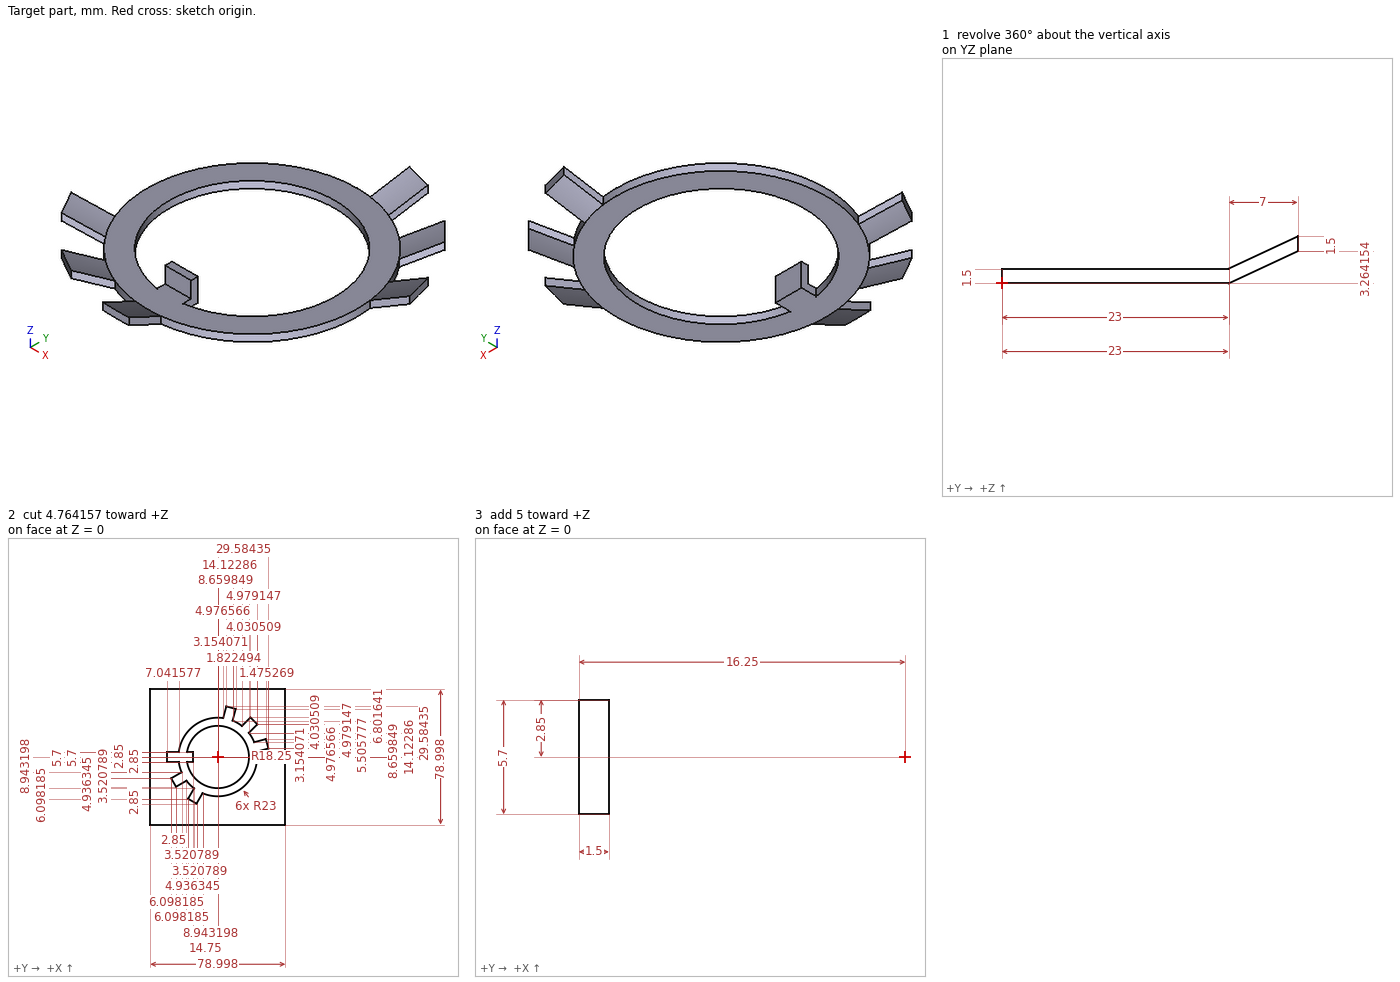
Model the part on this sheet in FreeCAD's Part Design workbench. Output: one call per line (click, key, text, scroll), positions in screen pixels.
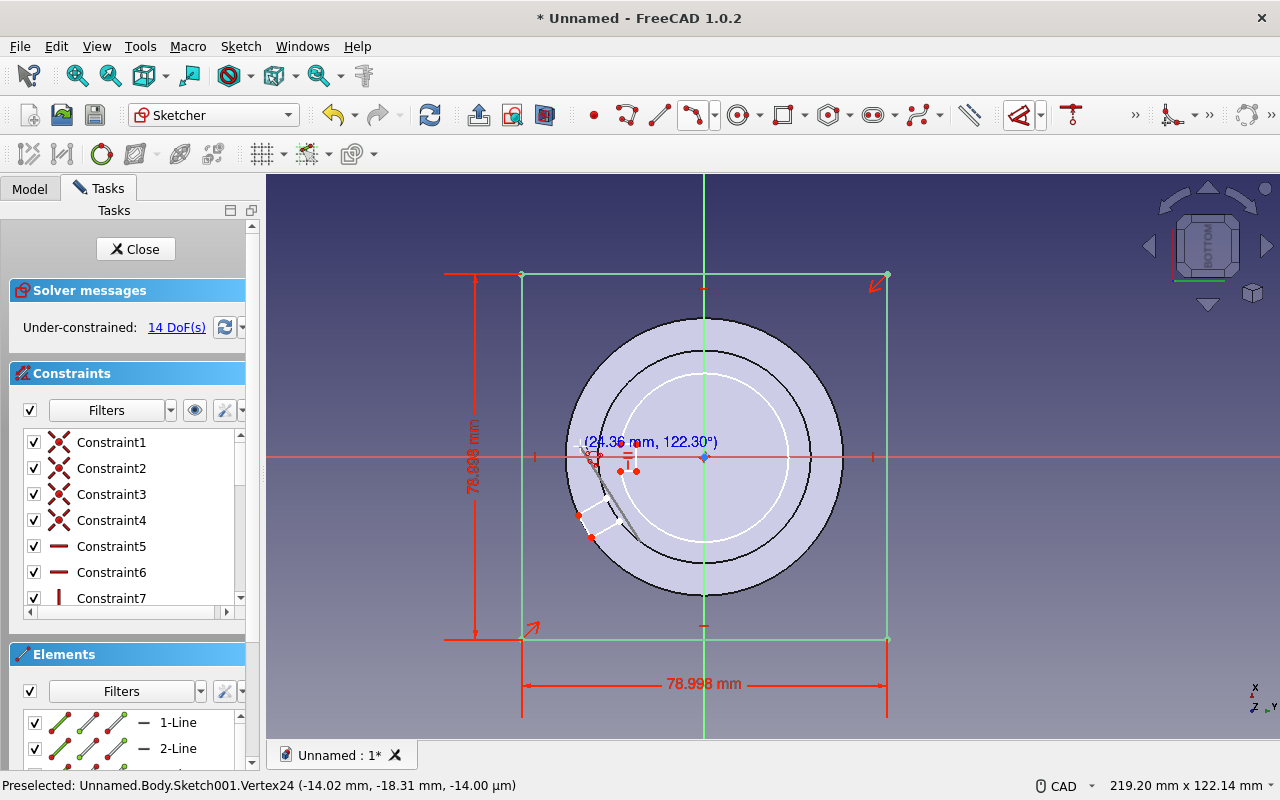
click(624, 570)
click(647, 583)
click(663, 555)
right_click(663, 555)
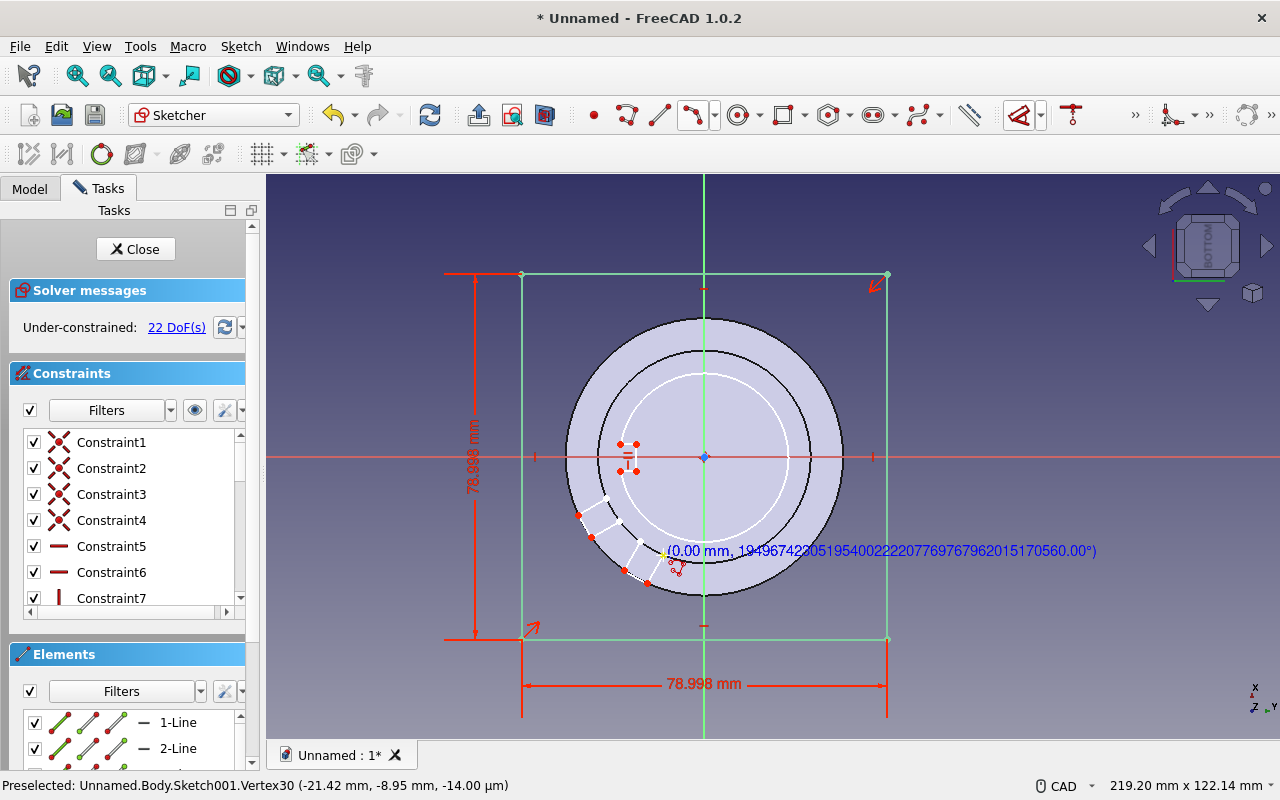
click(810, 442)
click(841, 434)
click(834, 408)
click(803, 417)
right_click(803, 417)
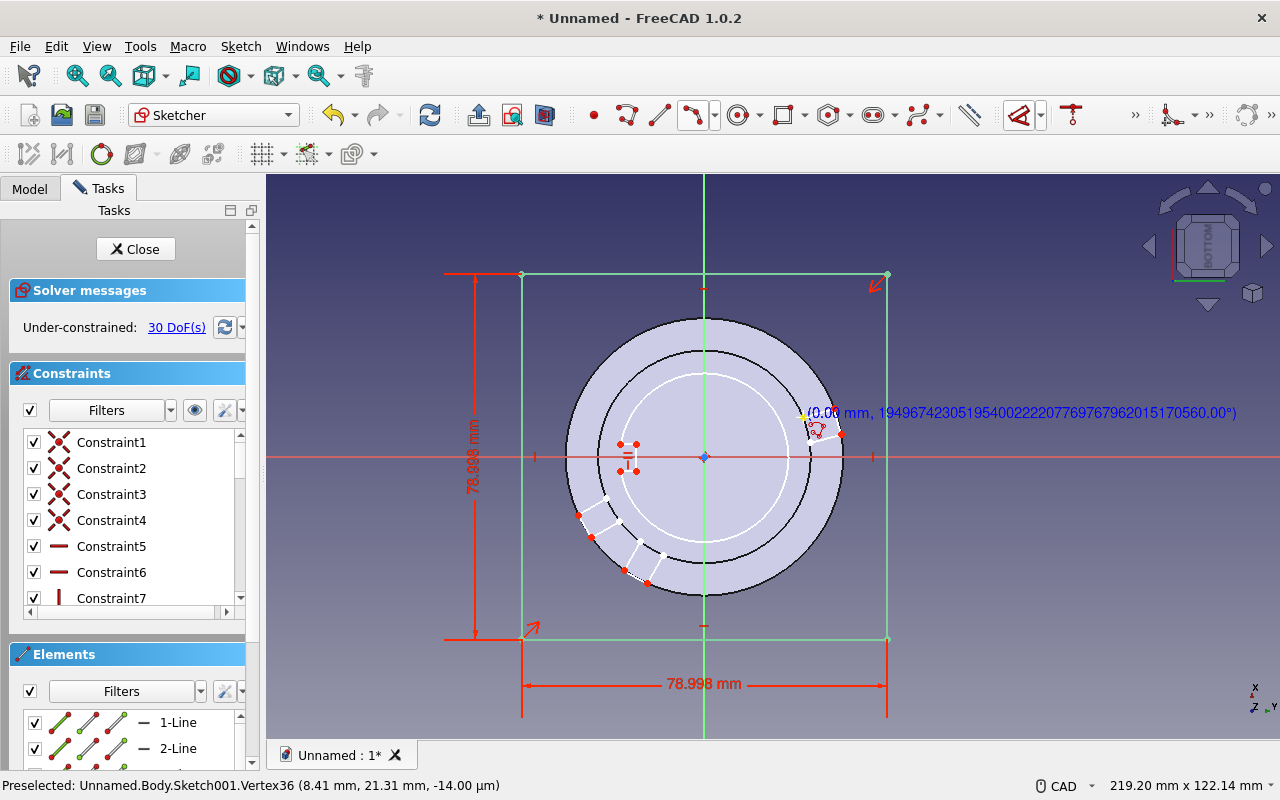
click(788, 392)
click(811, 369)
click(793, 350)
click(770, 373)
right_click(770, 373)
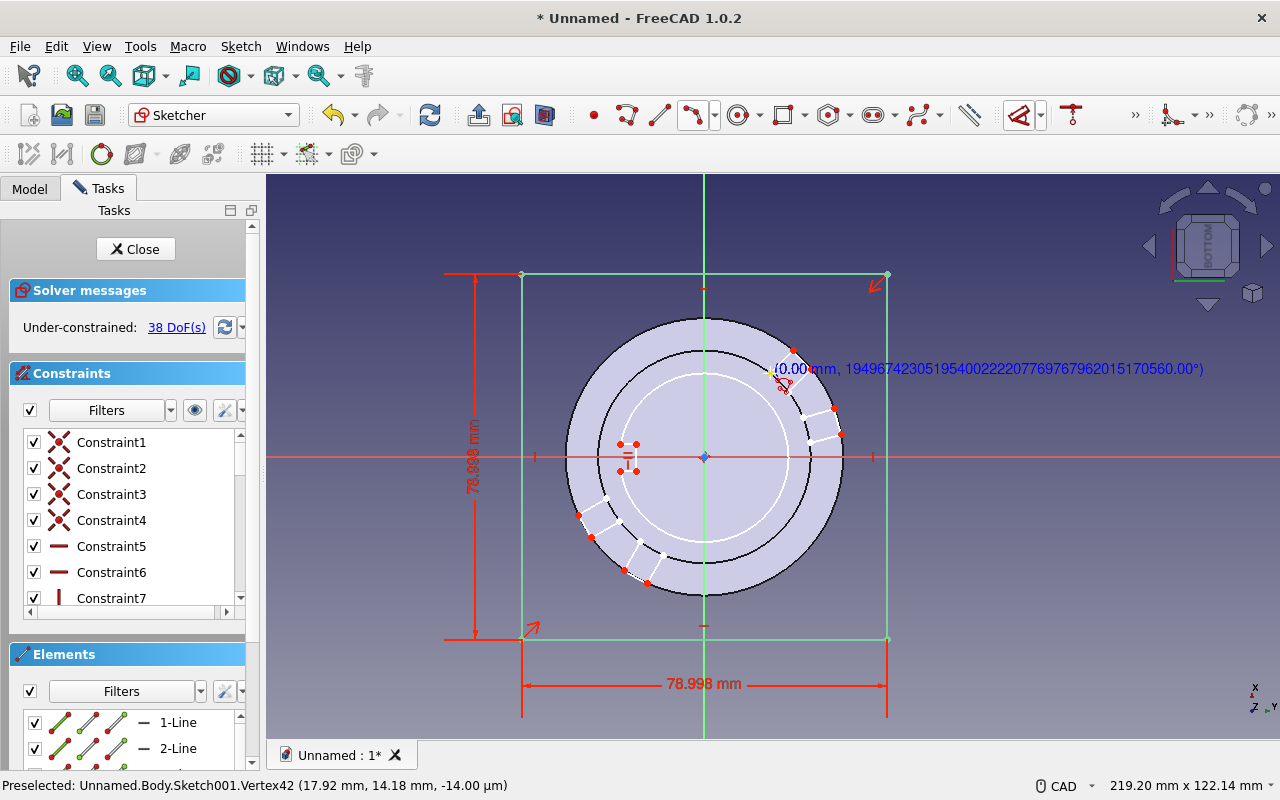
click(744, 358)
click(753, 327)
click(727, 320)
click(719, 352)
right_click(719, 352)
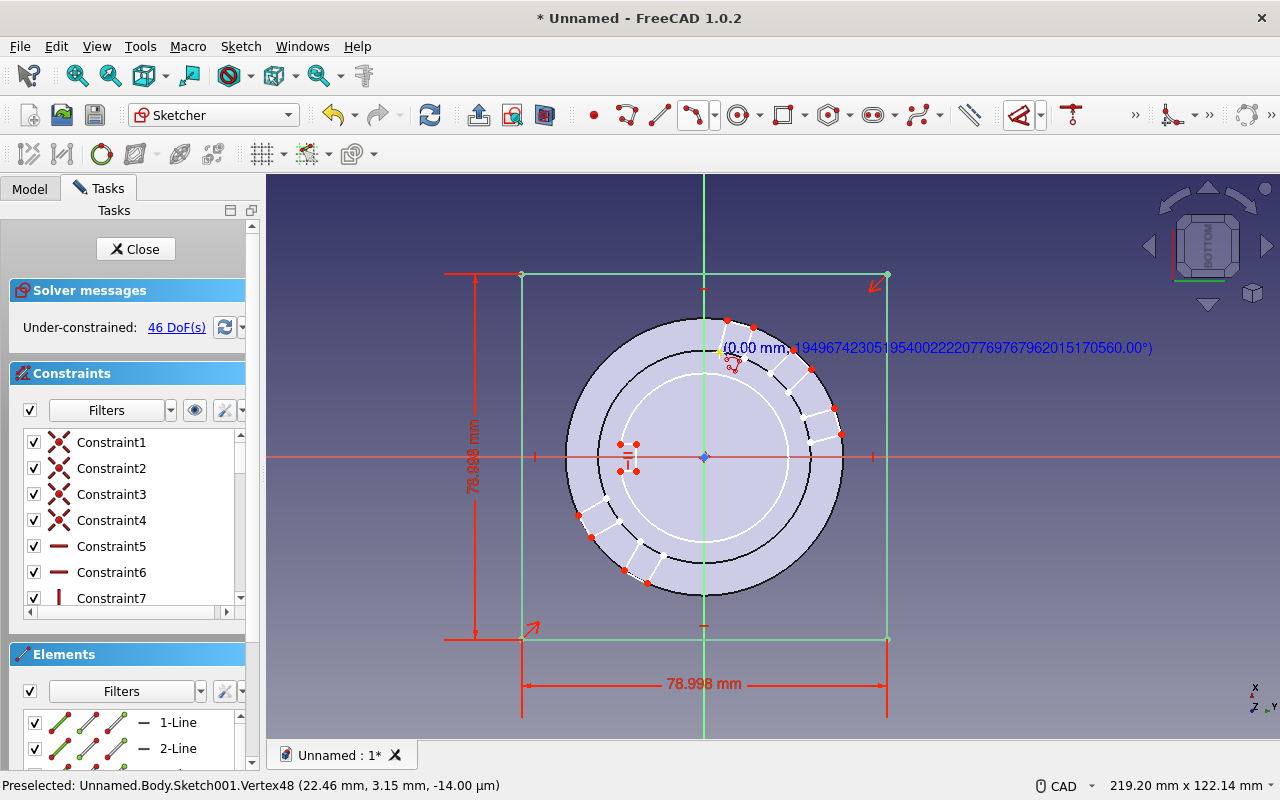
click(599, 444)
click(566, 444)
click(566, 470)
click(599, 470)
right_click(599, 470)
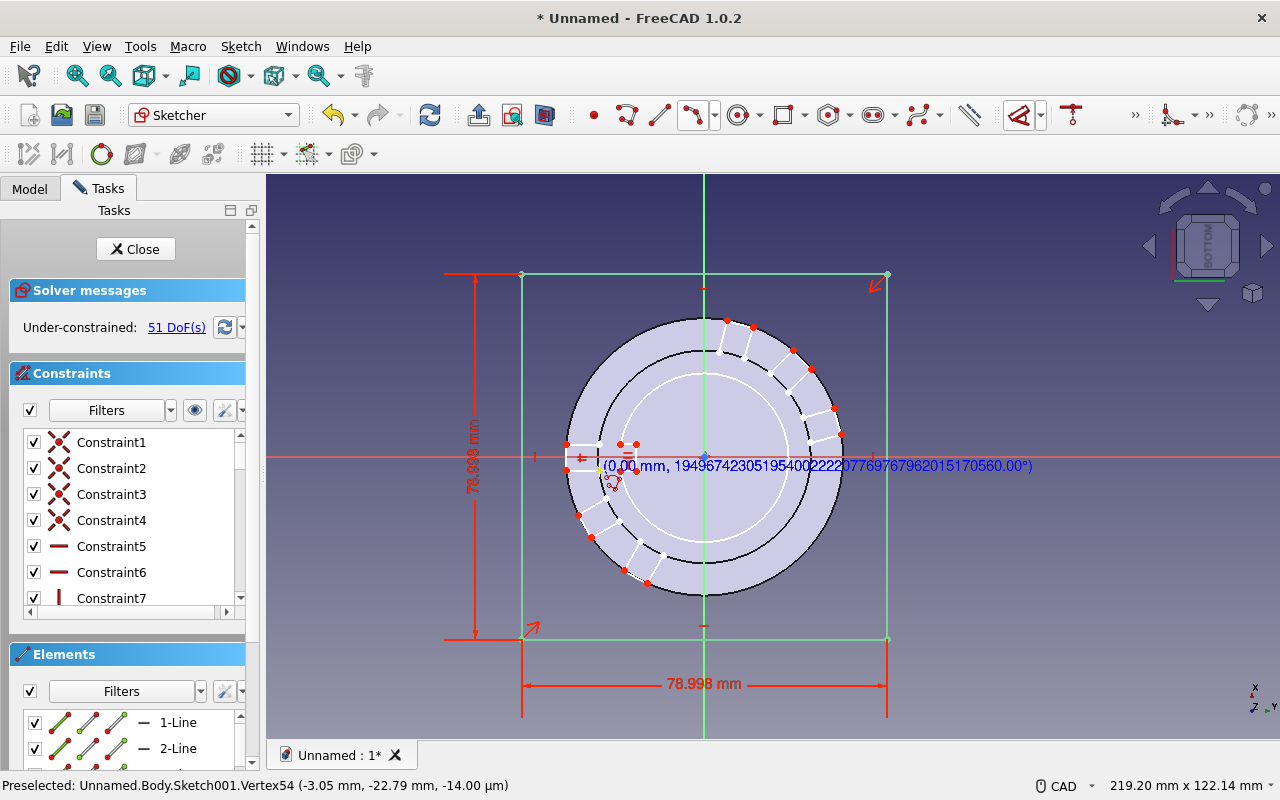
click(692, 116)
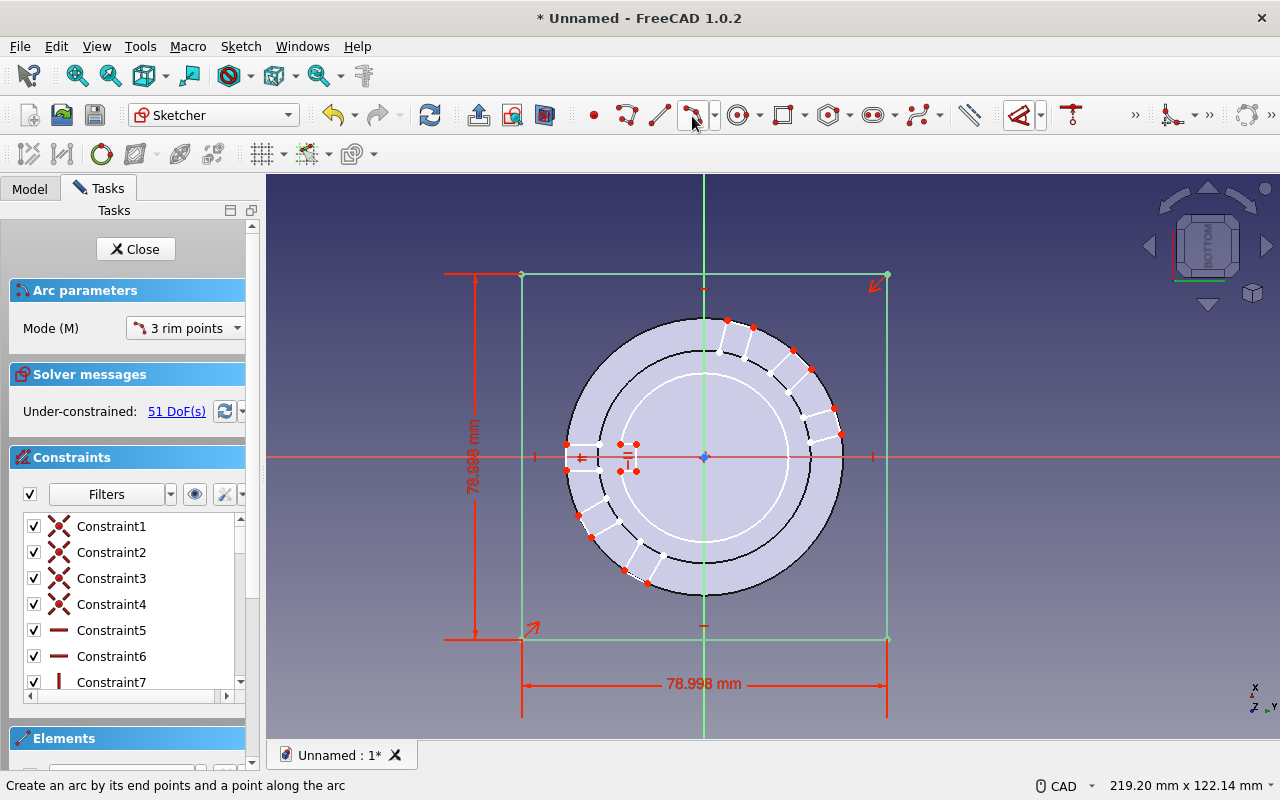
click(620, 522)
click(640, 542)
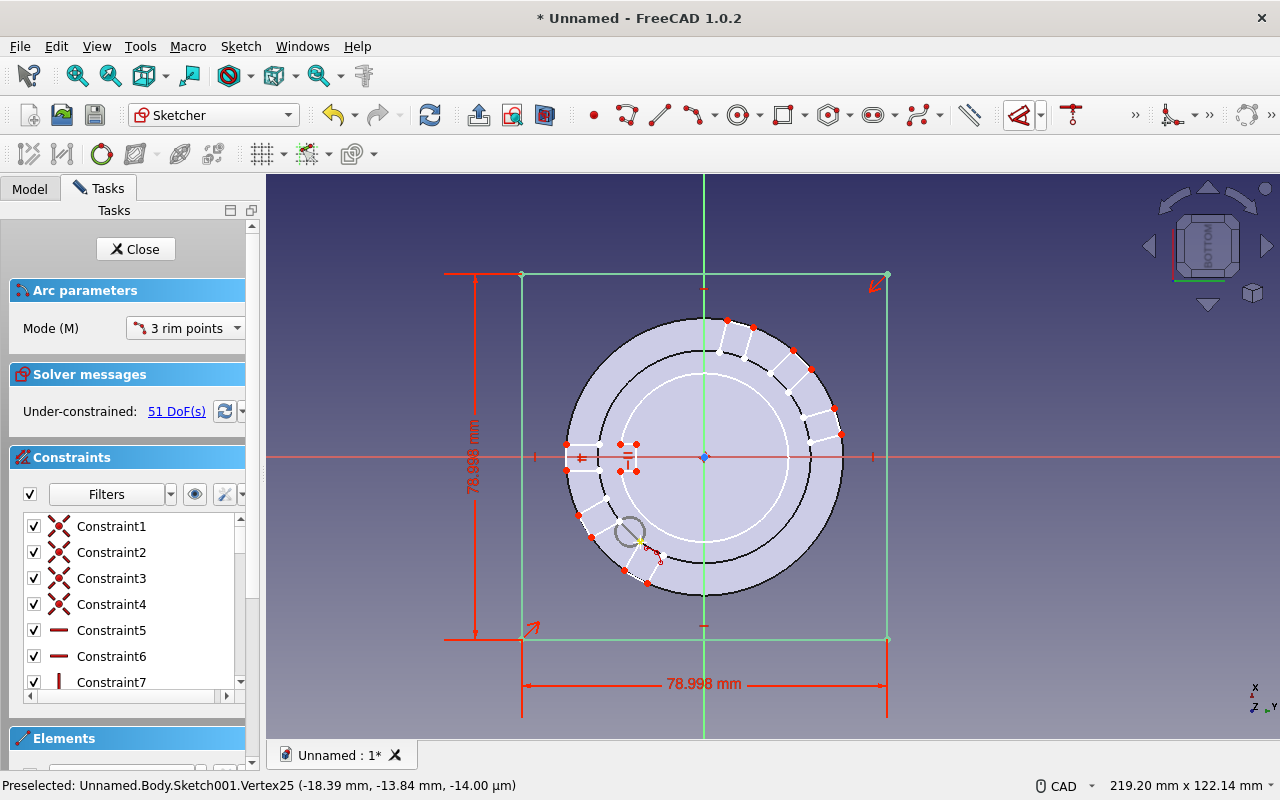
scroll(629, 532, up, 14)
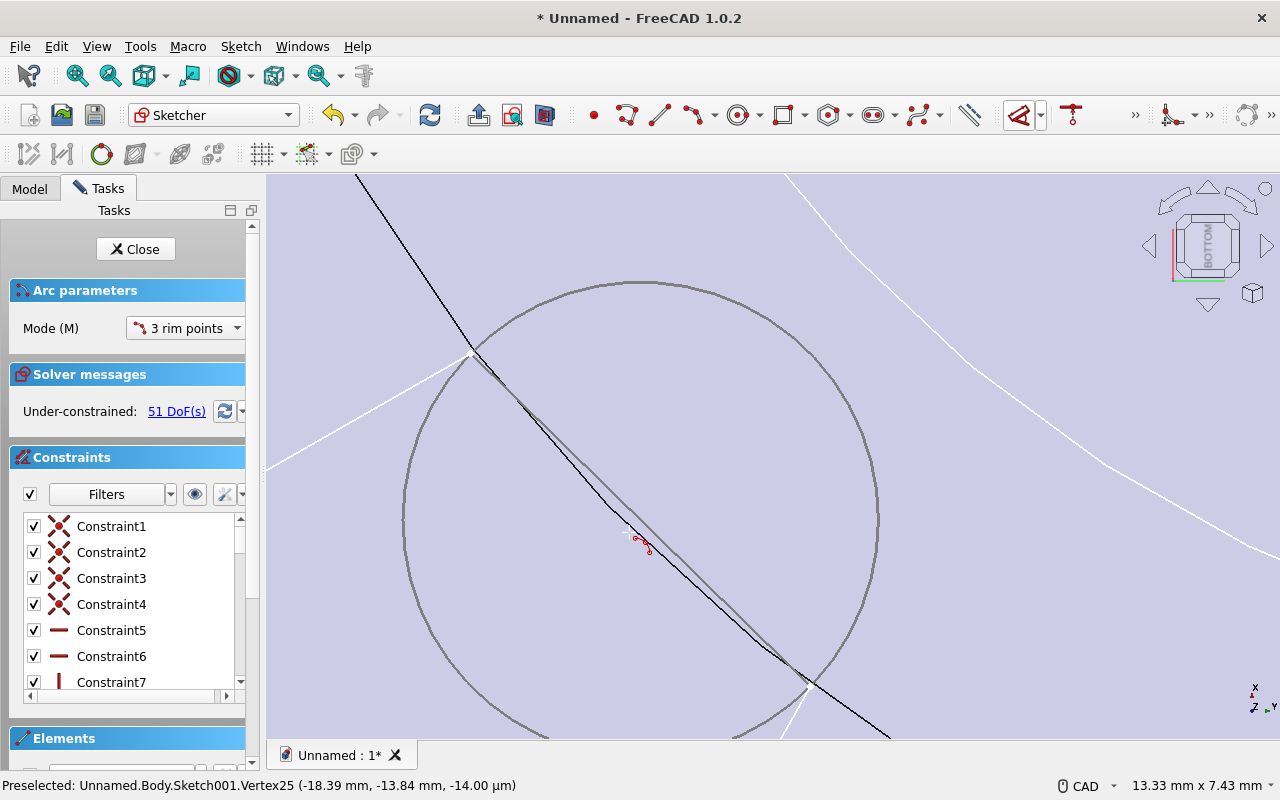
click(627, 524)